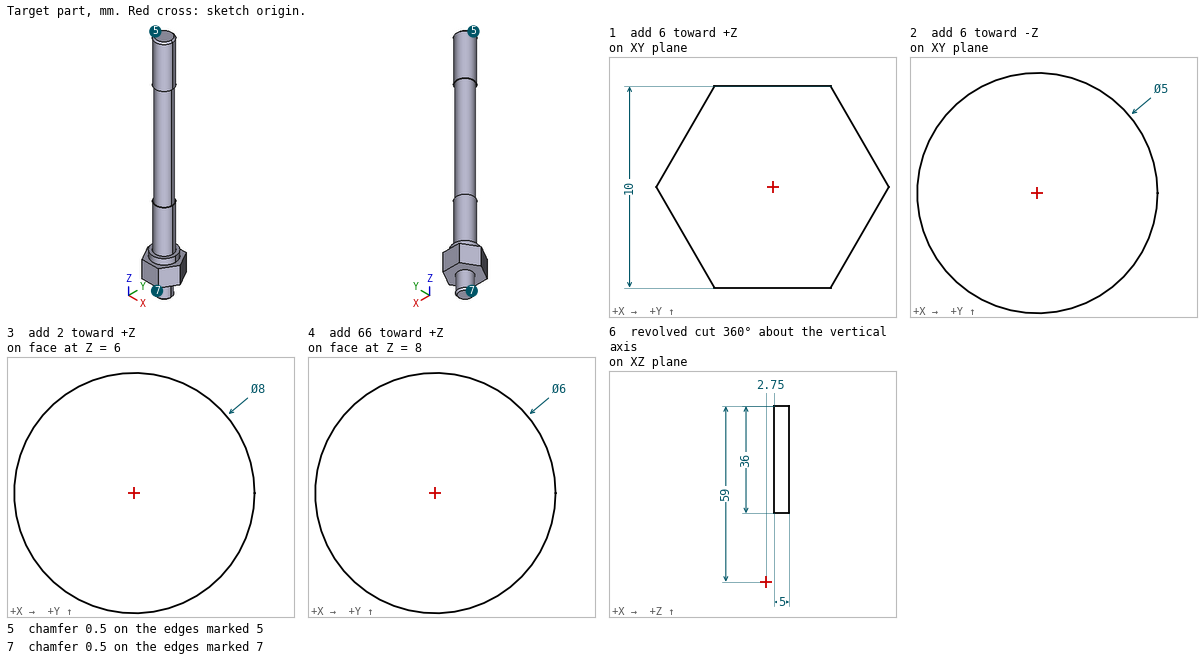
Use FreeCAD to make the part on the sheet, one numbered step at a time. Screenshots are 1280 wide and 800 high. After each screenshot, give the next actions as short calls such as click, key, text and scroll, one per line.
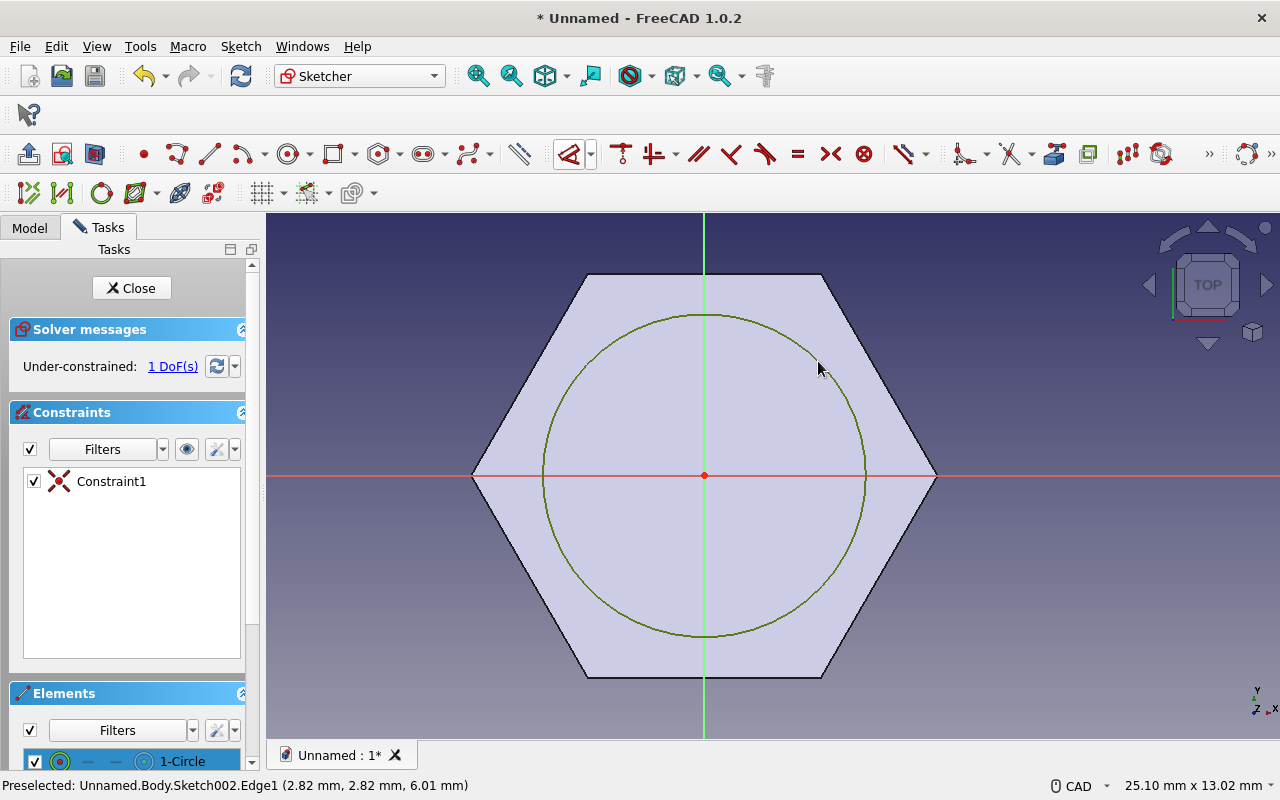
key(k)
key(o)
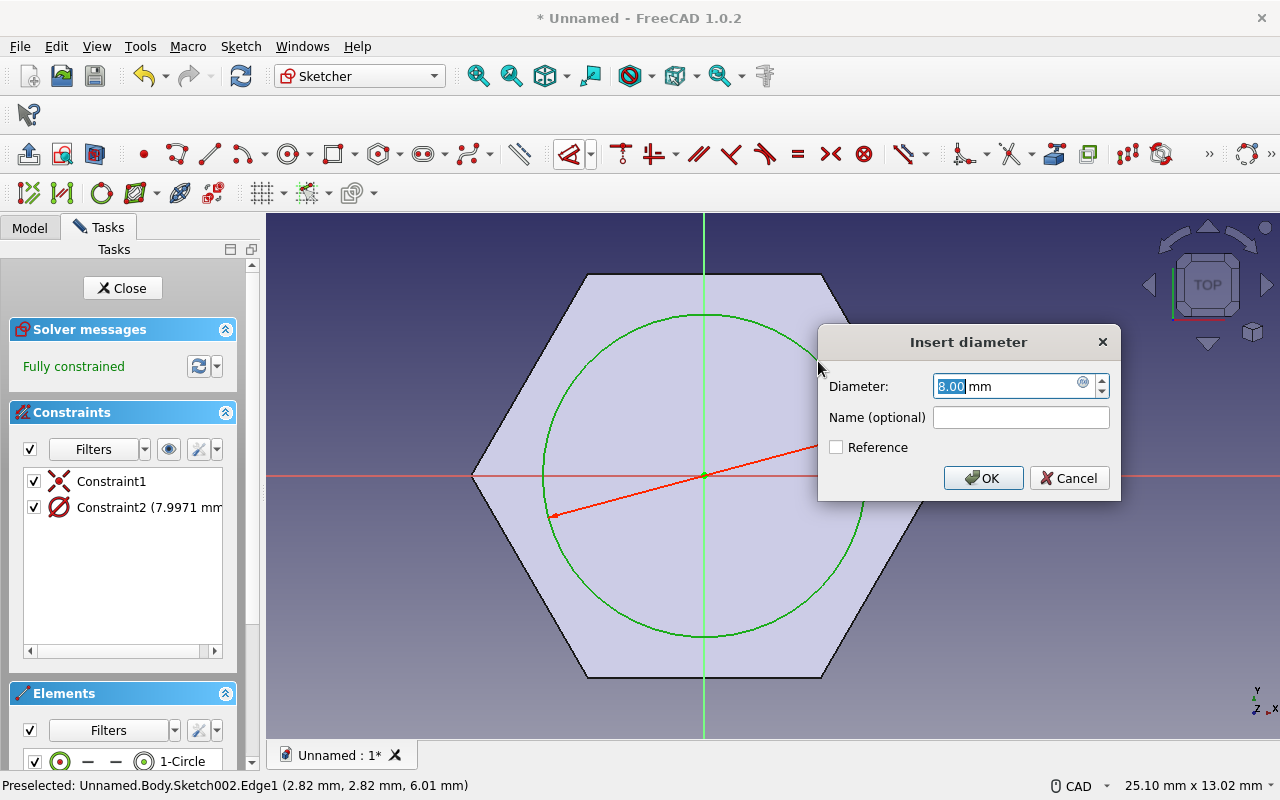
text(8)
key(Return)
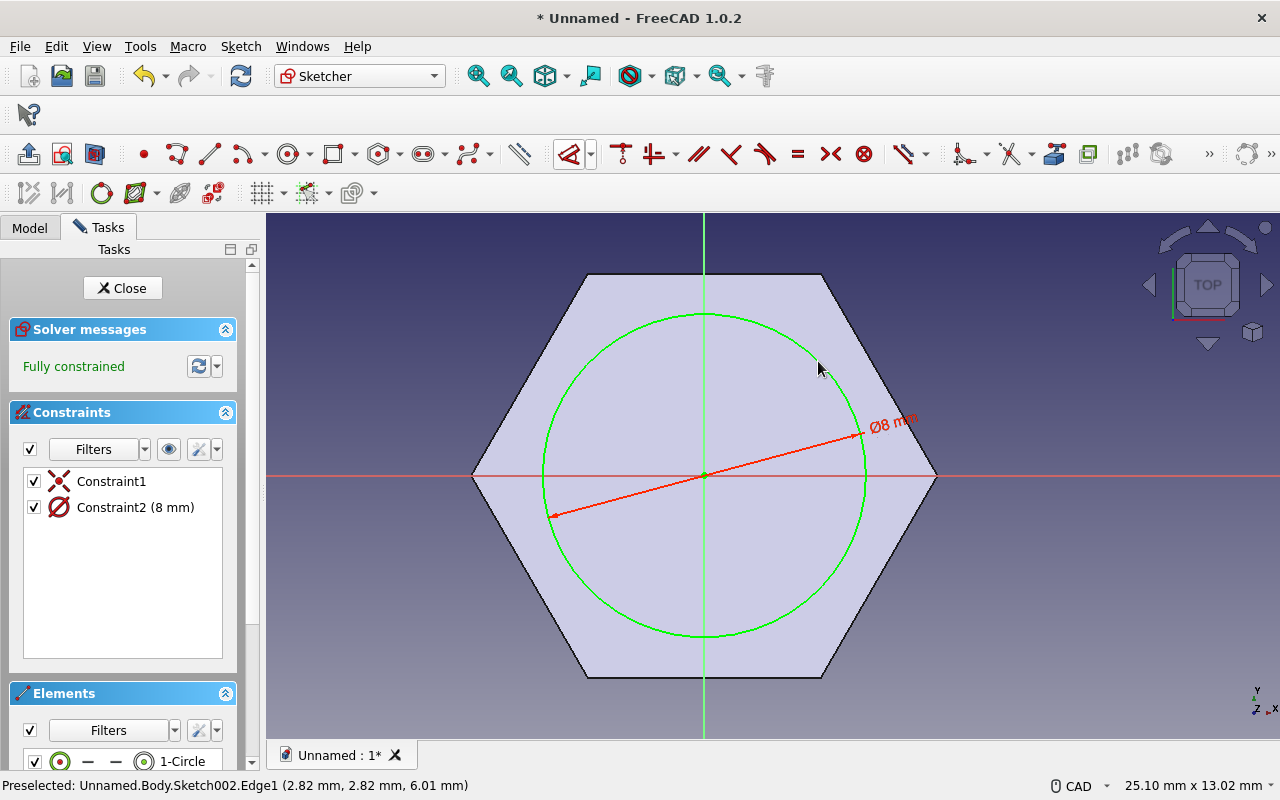
click(123, 288)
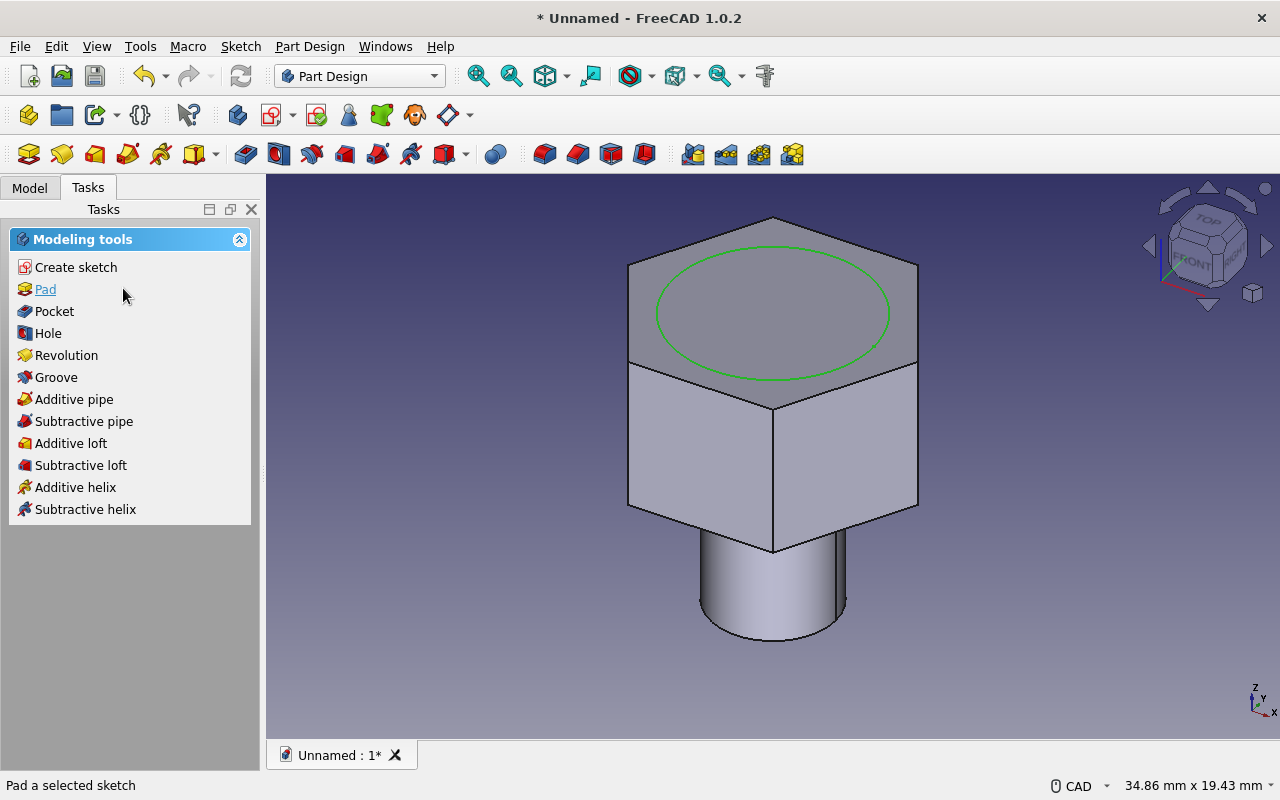
click(29, 154)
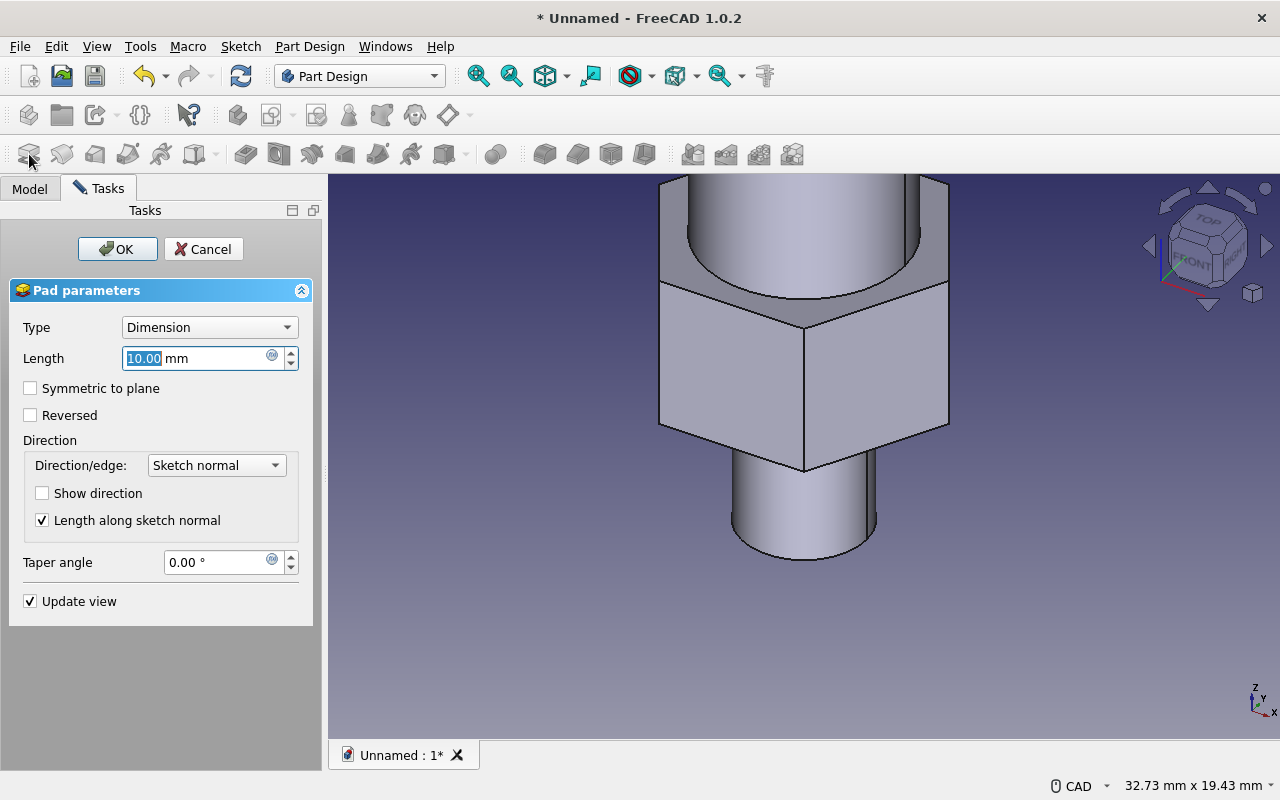
text(2)
key(Tab)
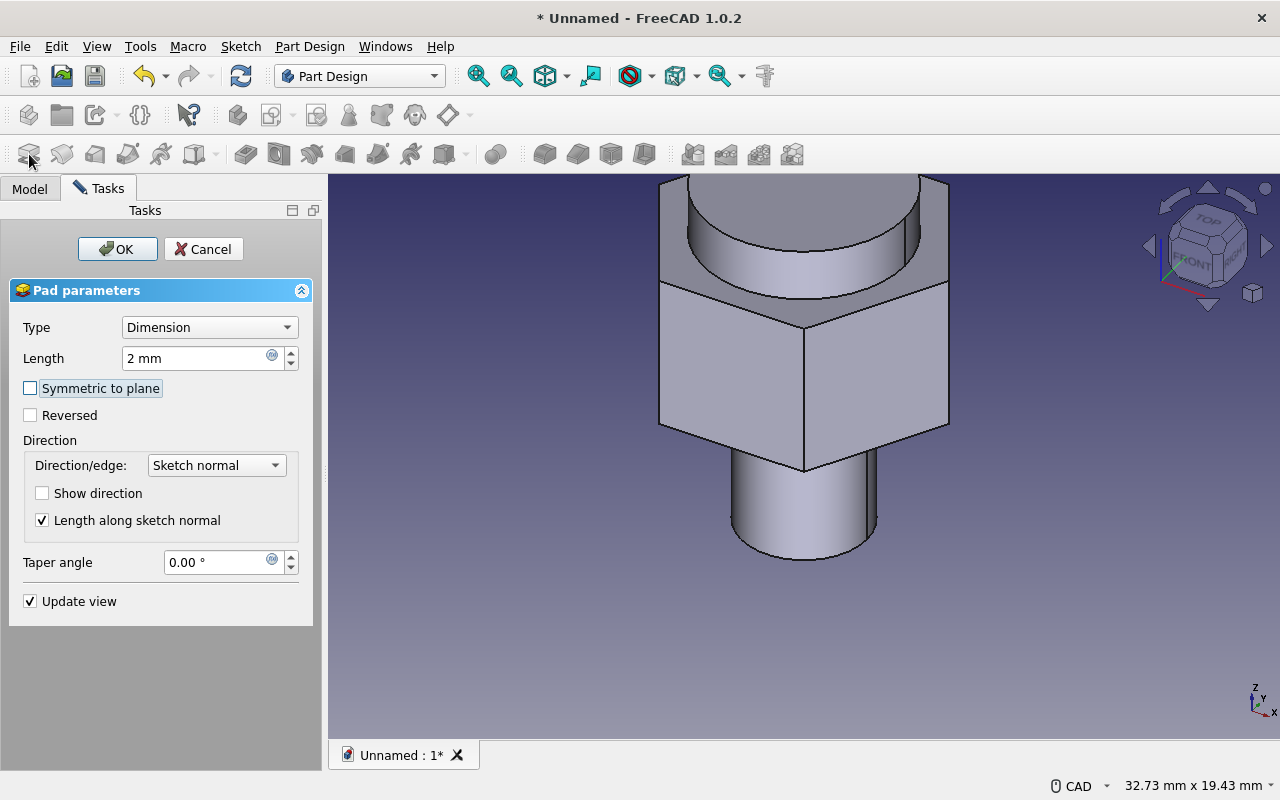
click(118, 249)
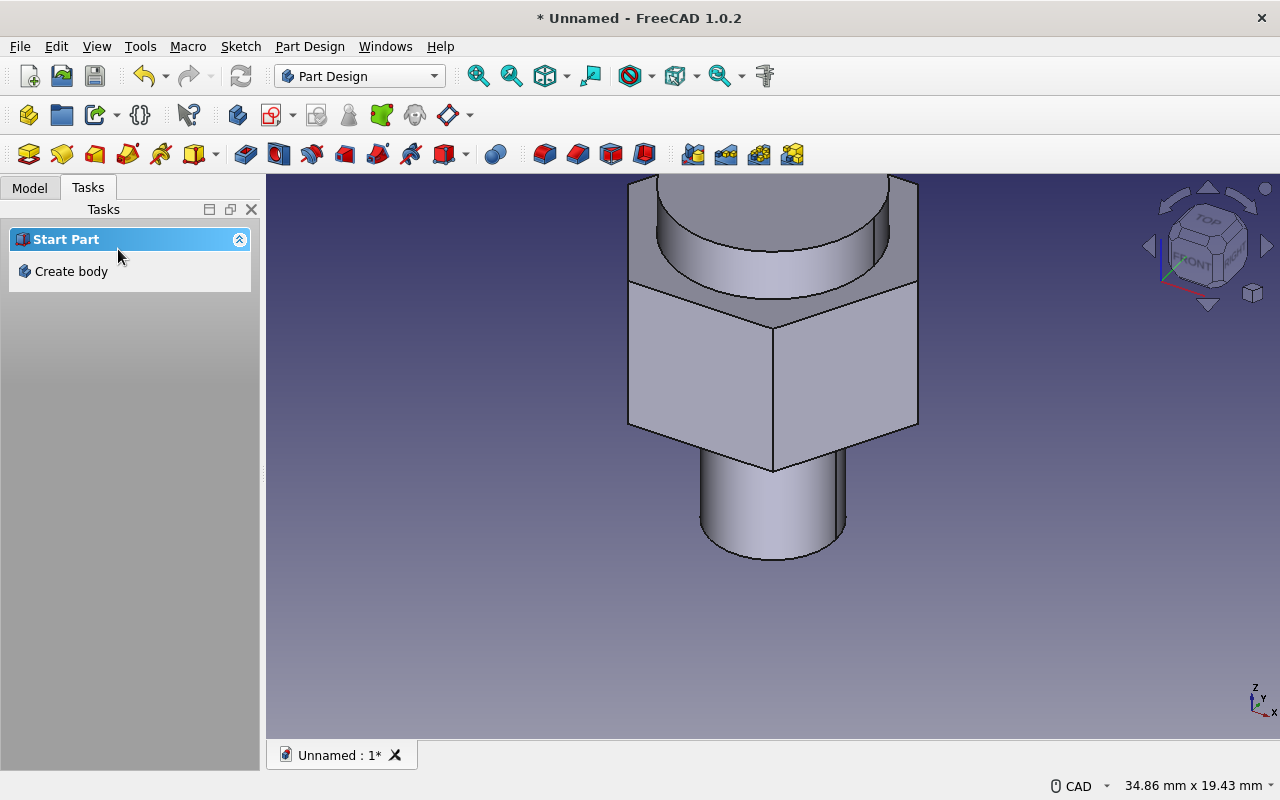
click(479, 76)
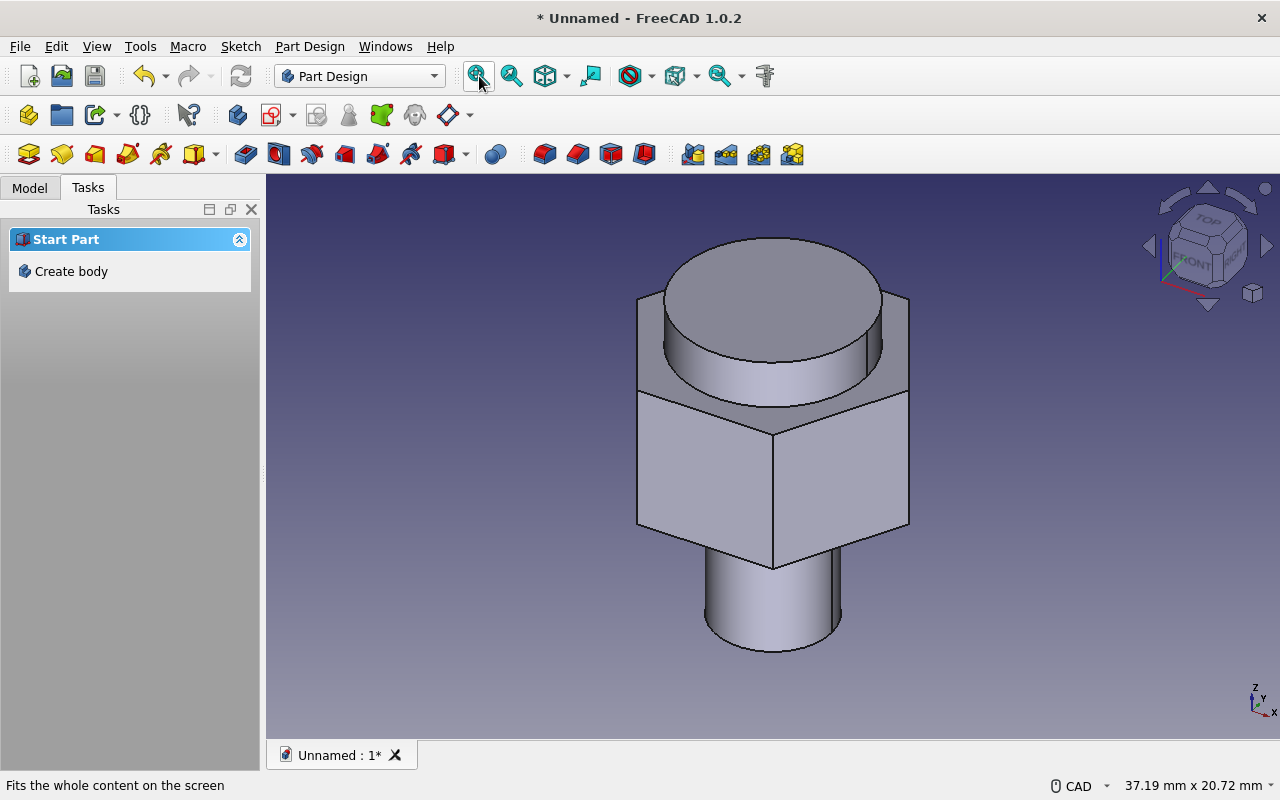
click(773, 299)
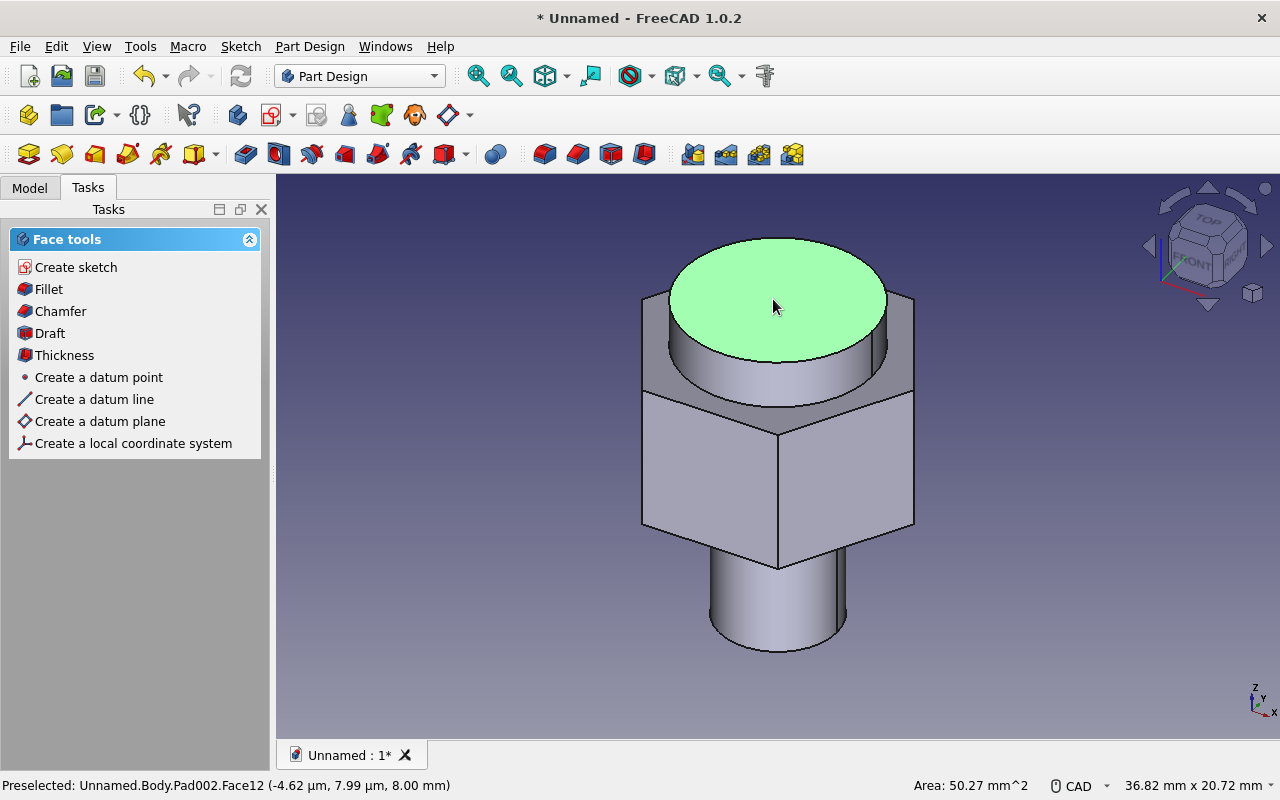
click(270, 116)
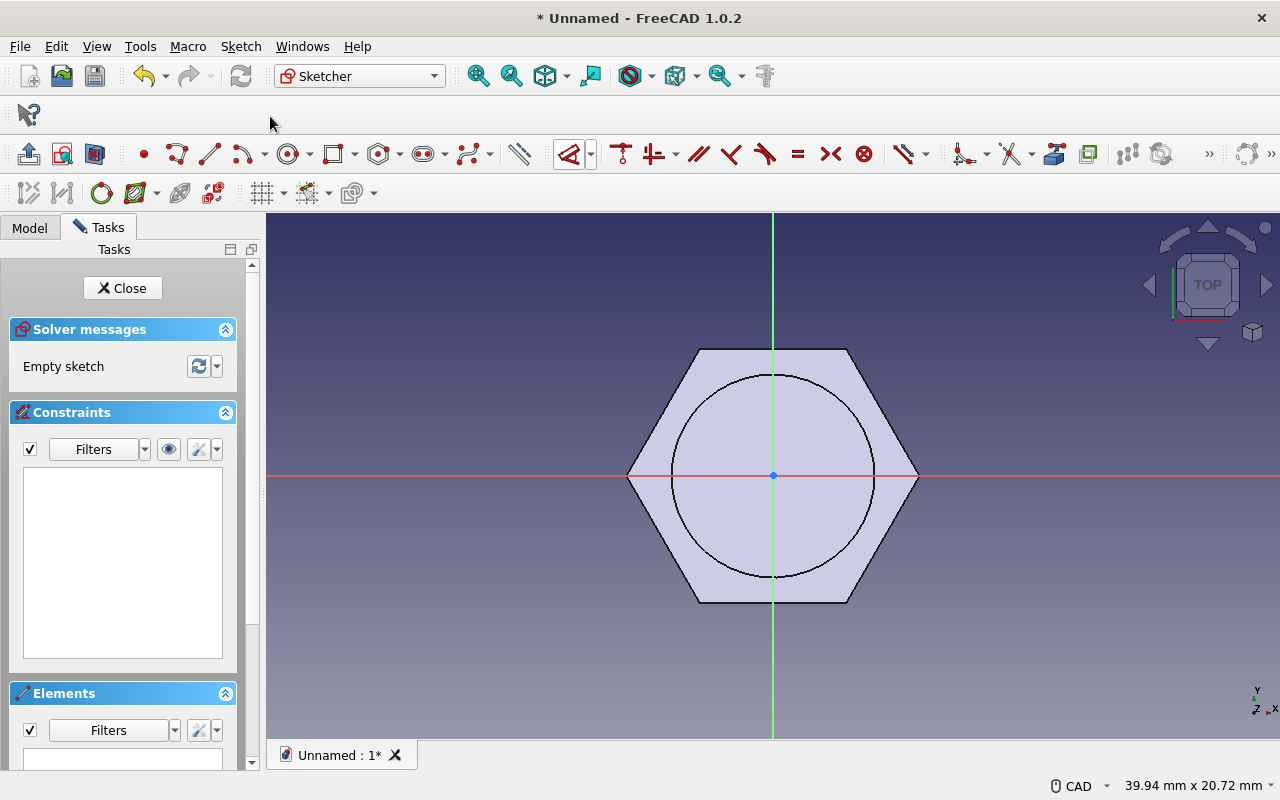
scroll(829, 476, up, 4)